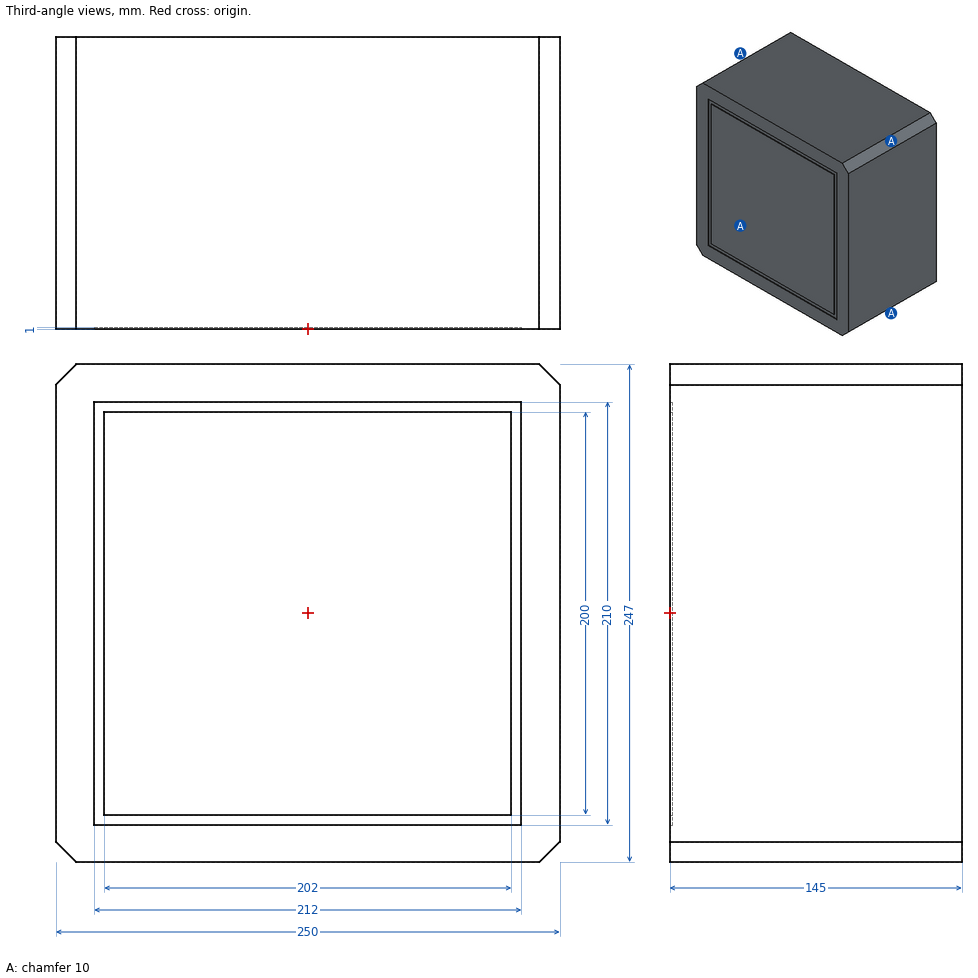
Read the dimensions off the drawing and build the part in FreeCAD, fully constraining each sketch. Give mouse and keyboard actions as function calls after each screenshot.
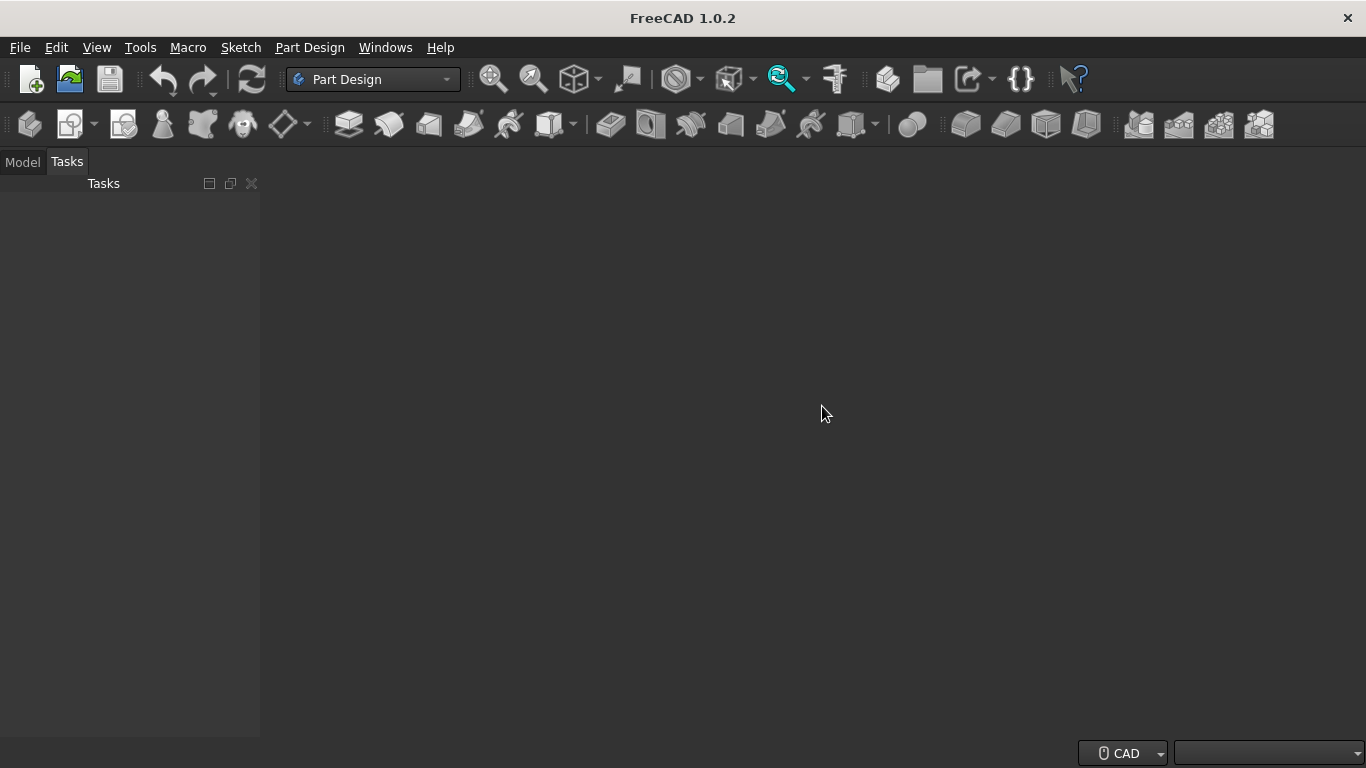
click(30, 80)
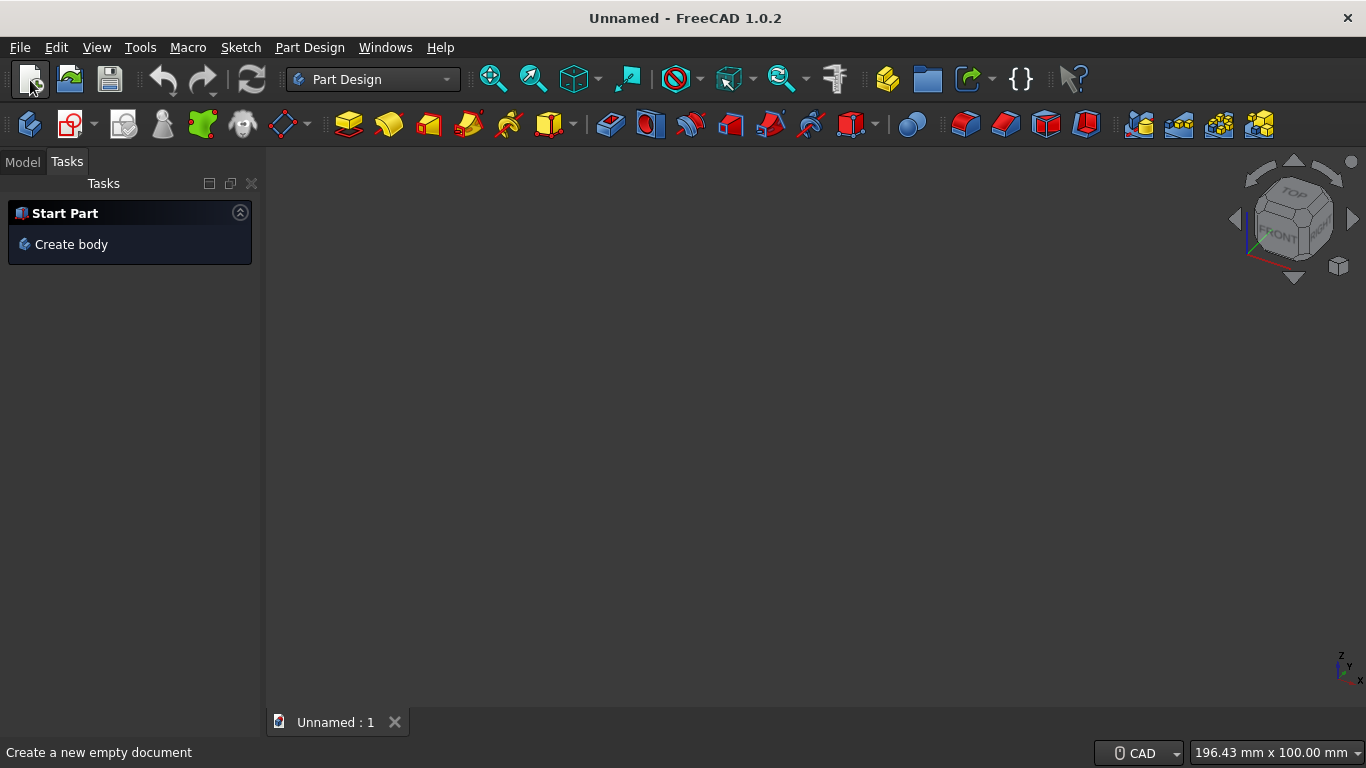
click(70, 124)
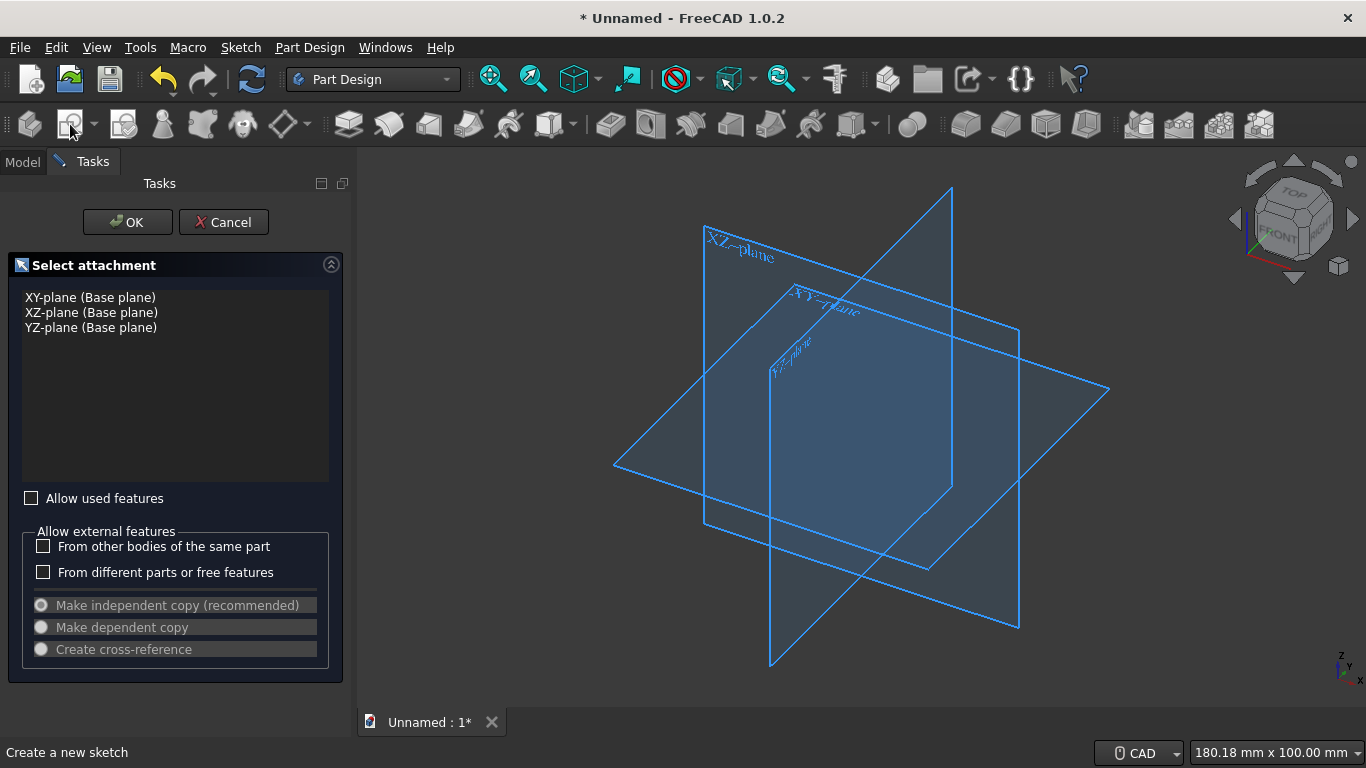
click(82, 312)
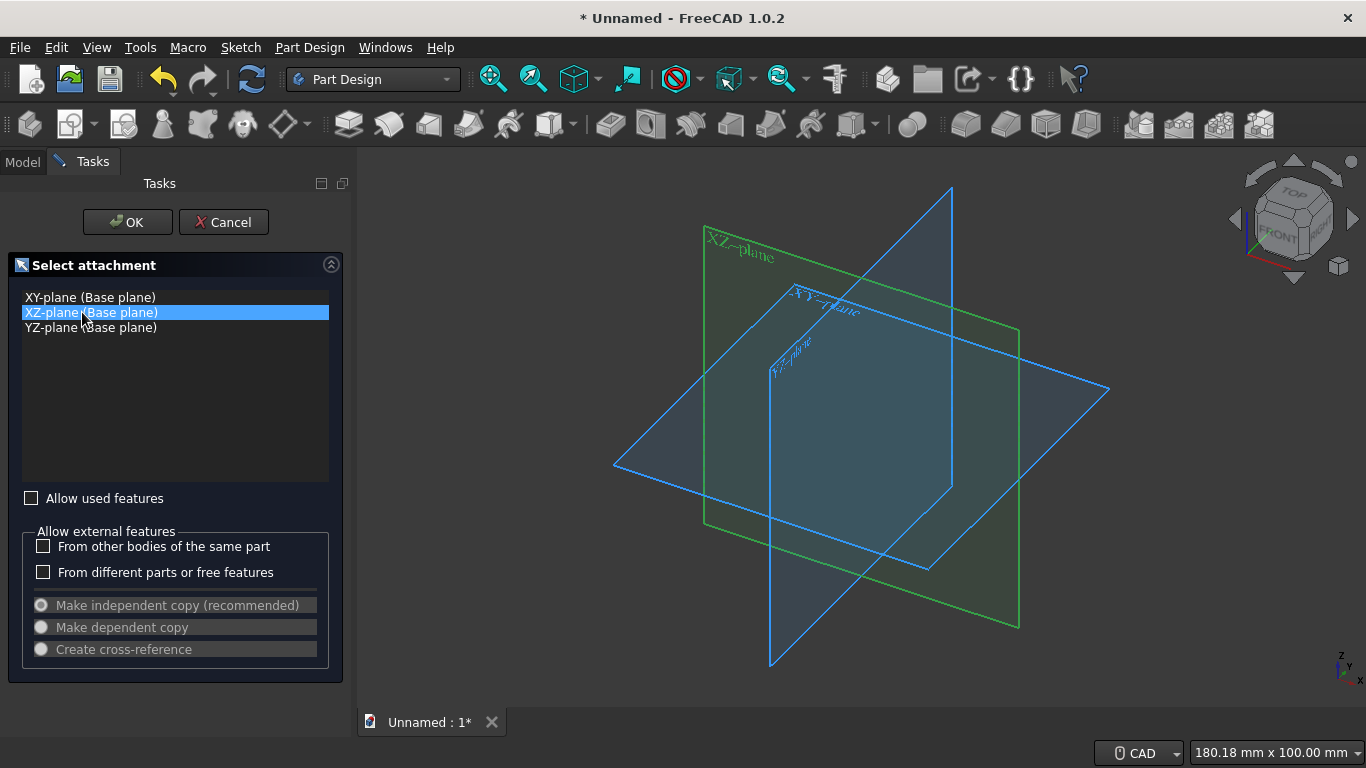
click(128, 222)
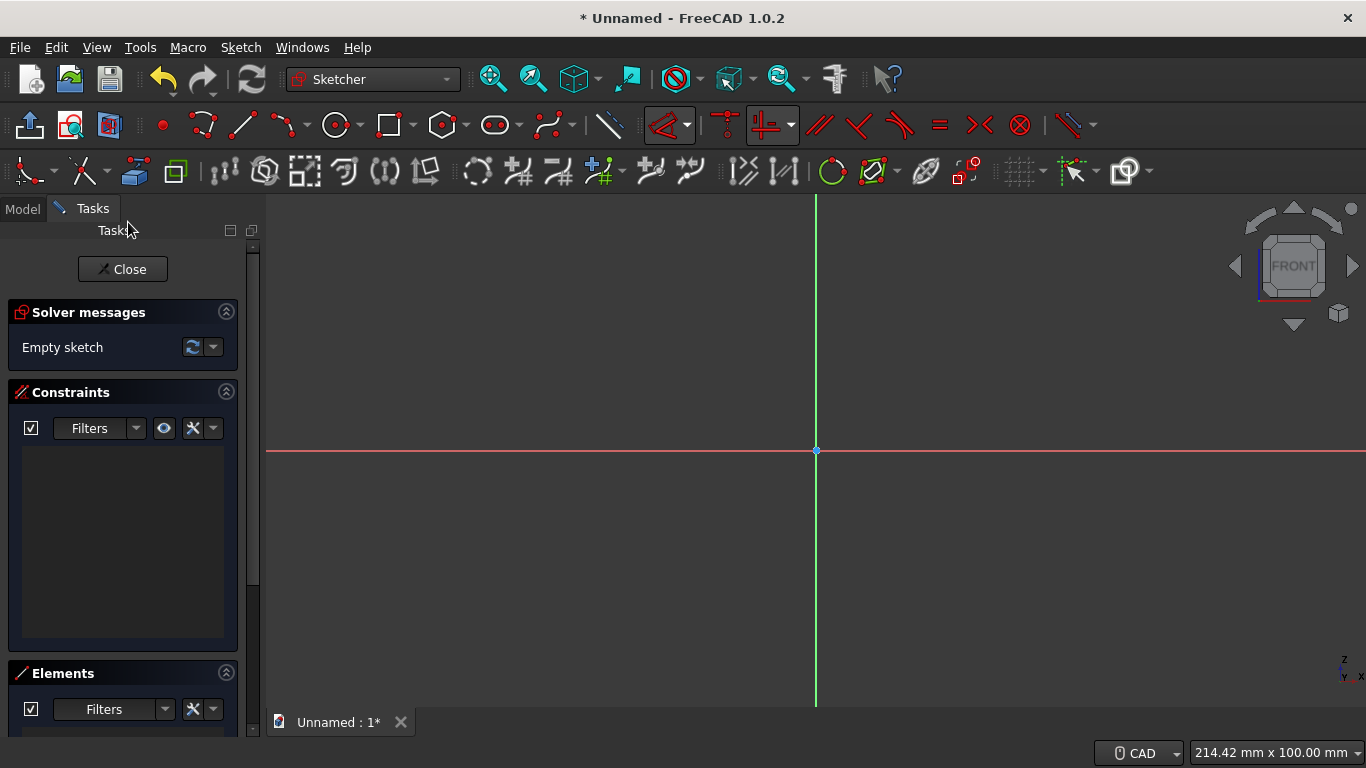
scroll(725, 451, down, 7)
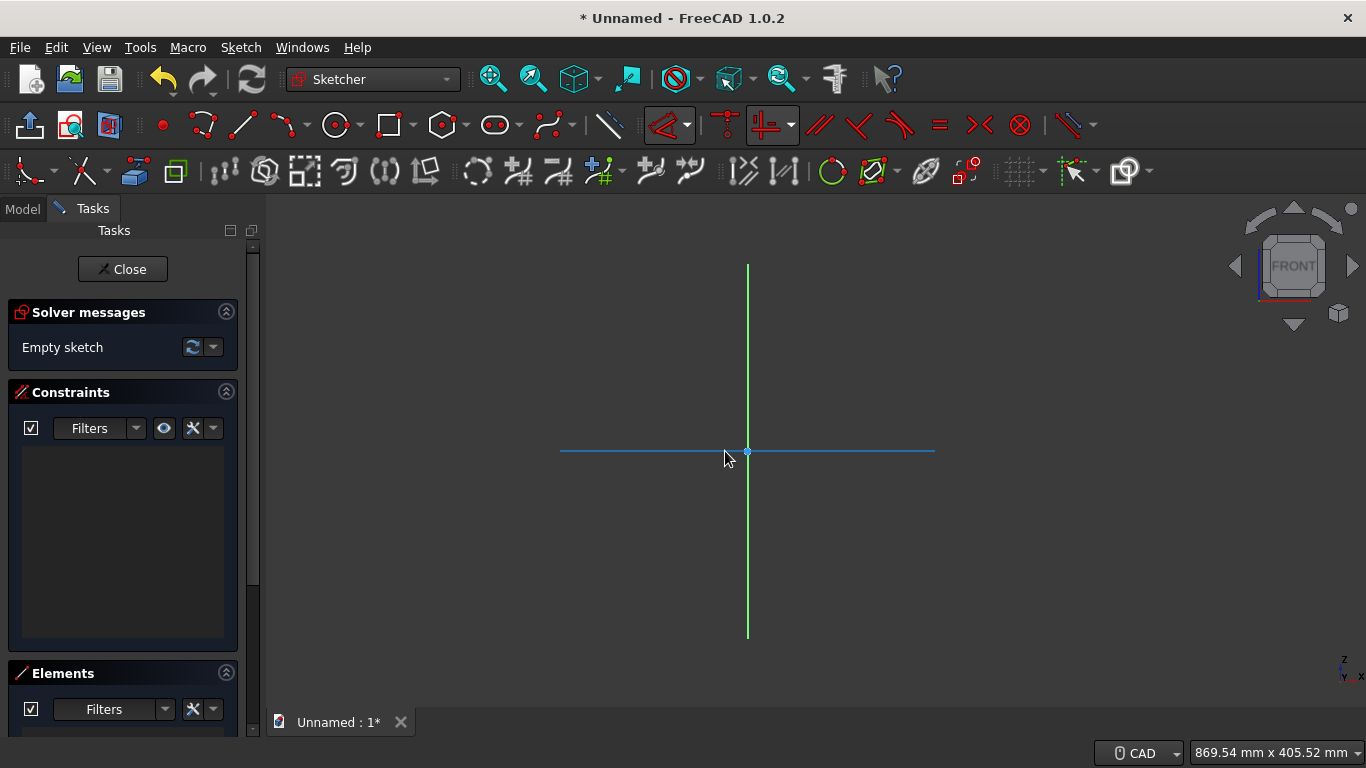
click(416, 126)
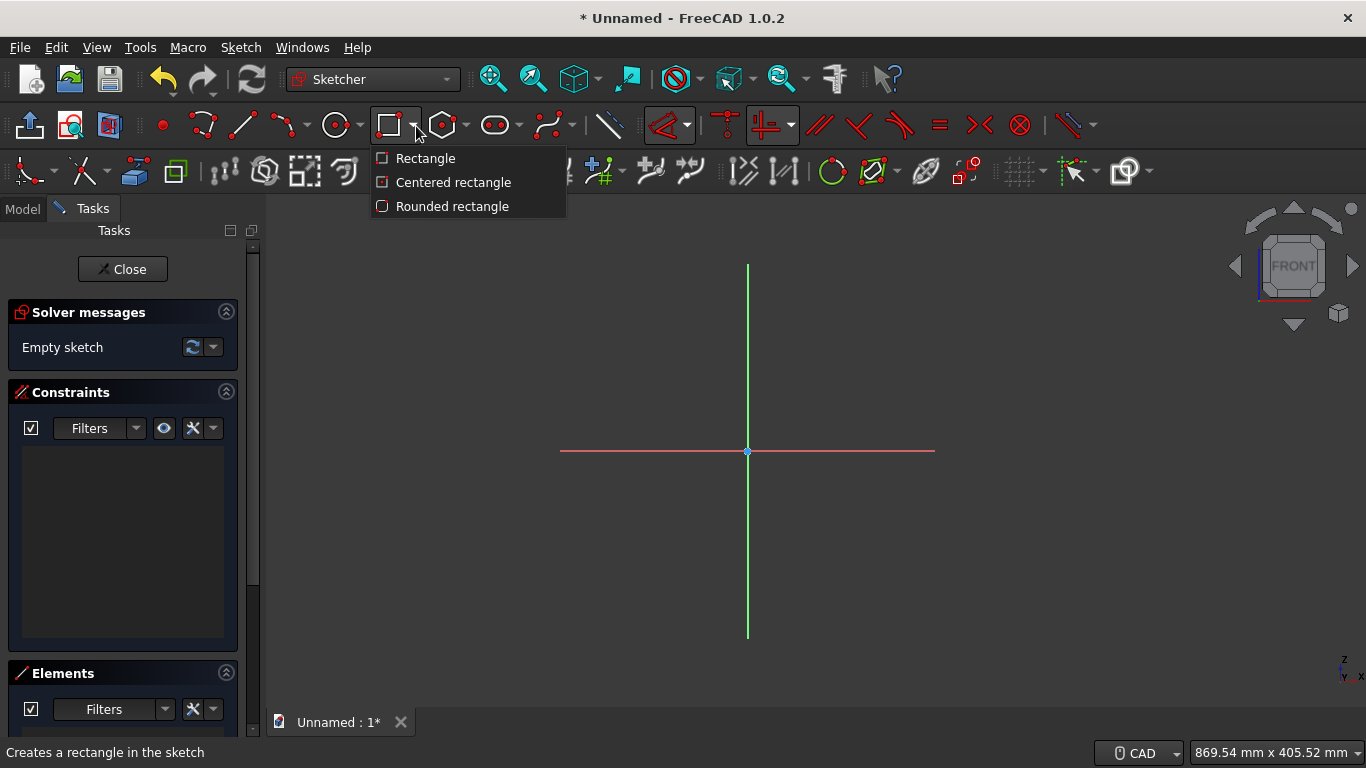
click(468, 182)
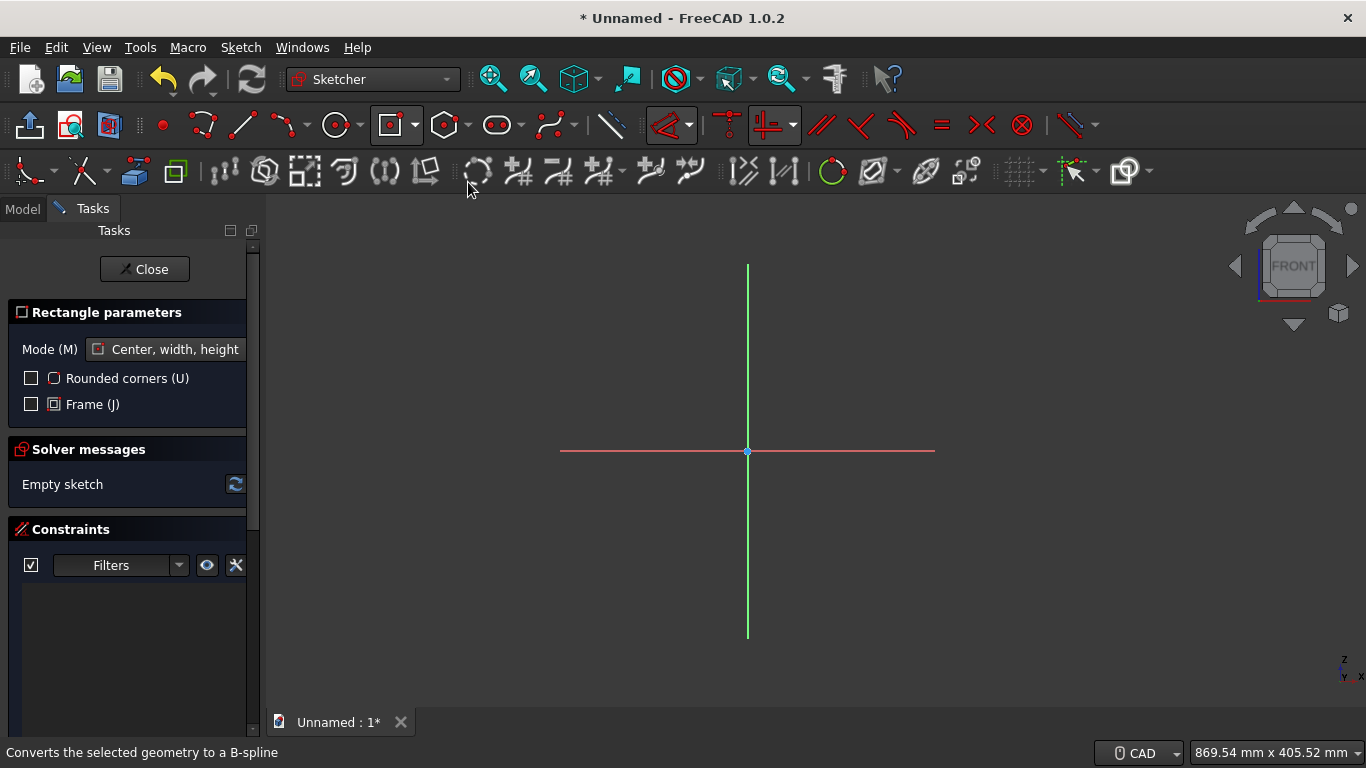
click(748, 451)
move(906, 295)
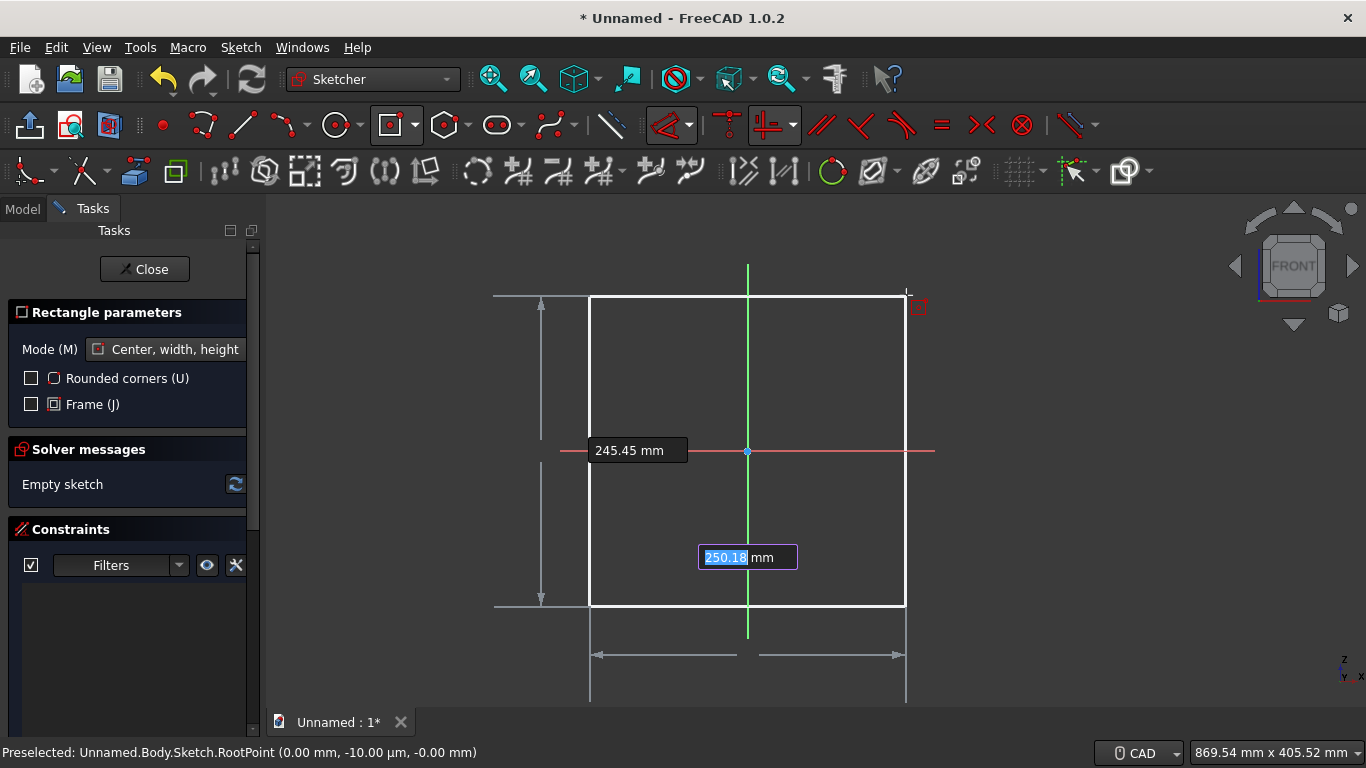
text(250)
key(Tab)
text(247)
key(Return)
key(Escape)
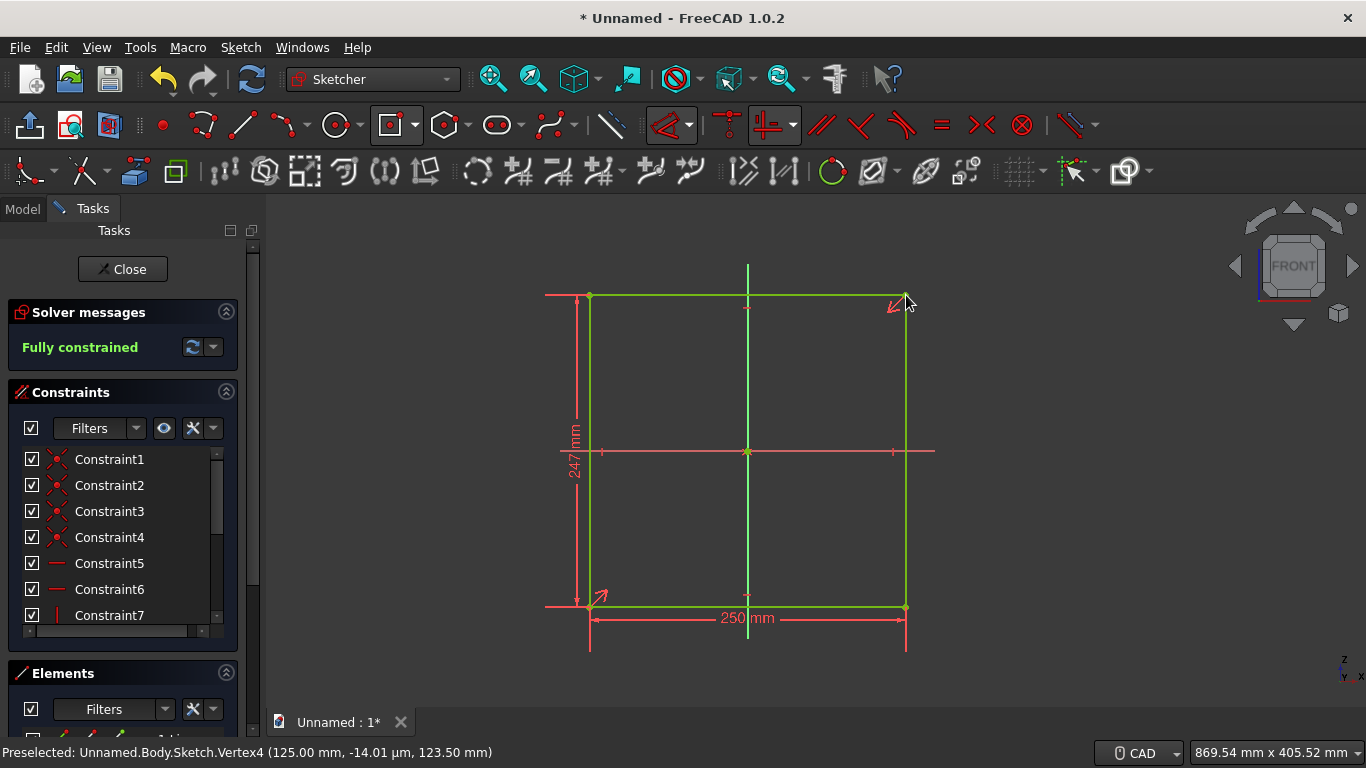
click(123, 269)